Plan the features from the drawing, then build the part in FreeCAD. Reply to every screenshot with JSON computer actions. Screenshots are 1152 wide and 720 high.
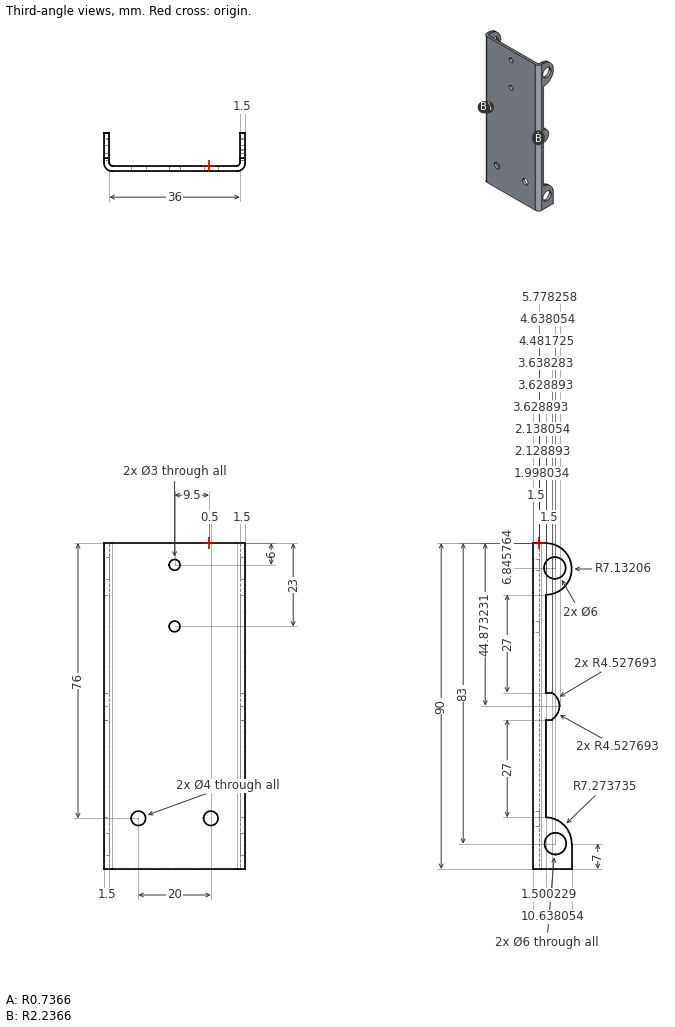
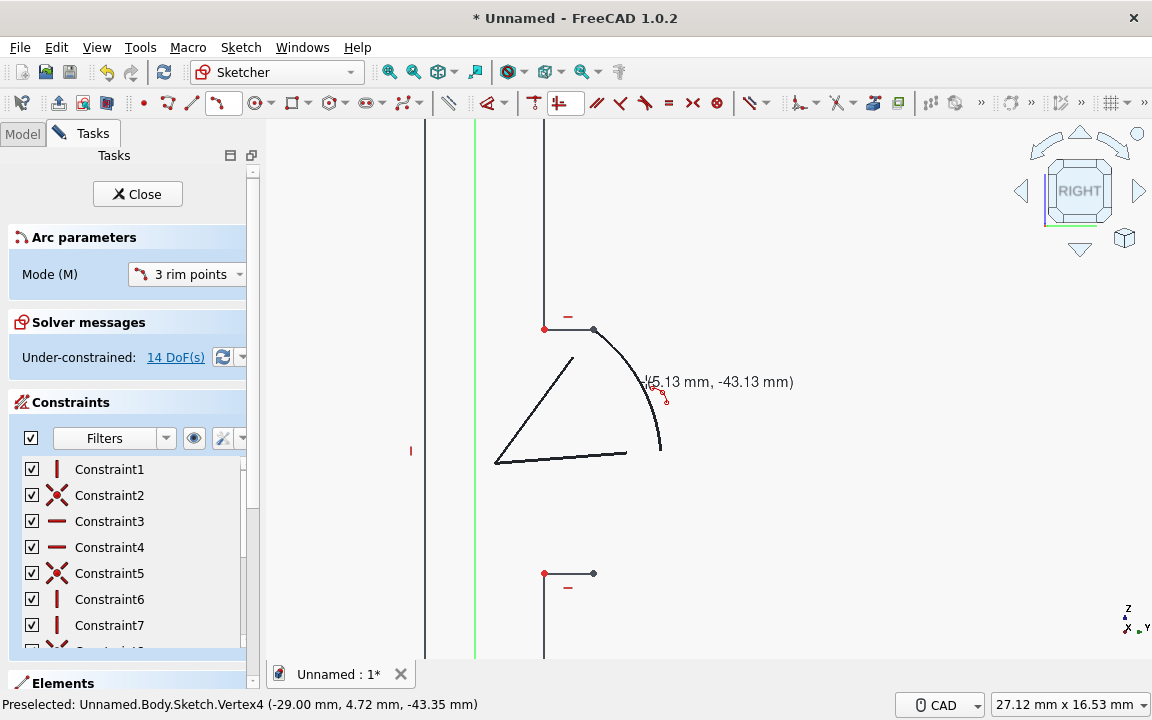
{"action": "left_click", "coordinate": [643, 376]}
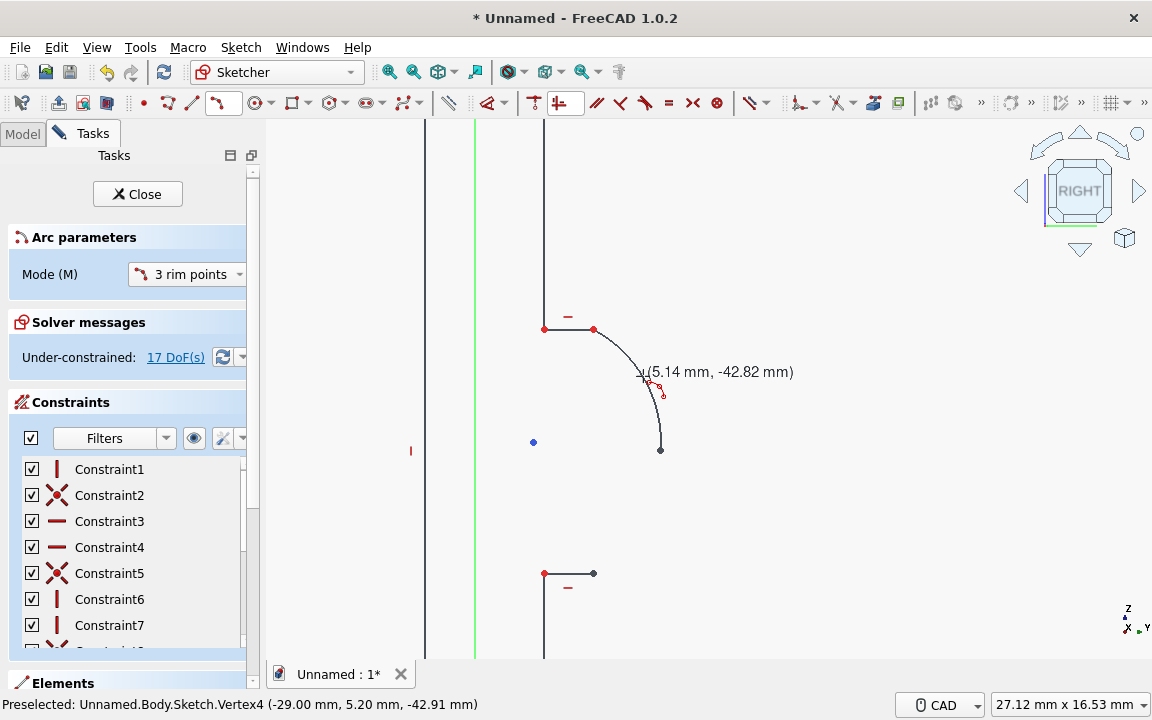
{"action": "scroll", "coordinate": [646, 382], "scroll_direction": "down", "scroll_amount": 11}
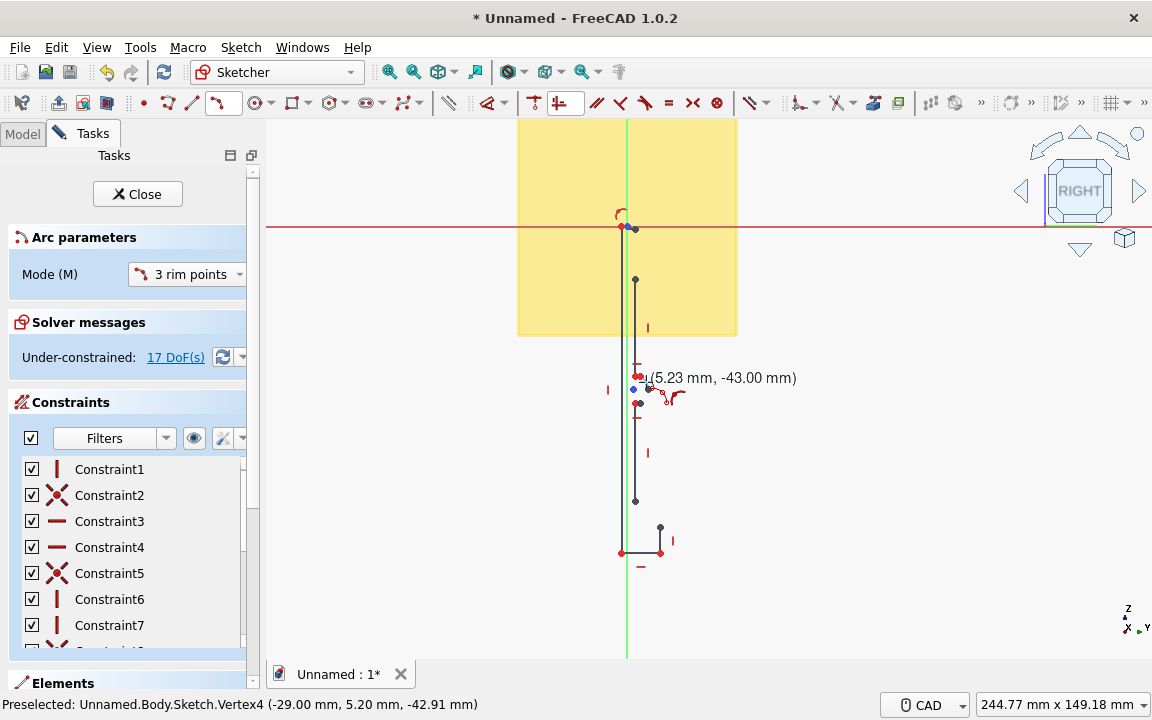
{"action": "left_click", "coordinate": [648, 390]}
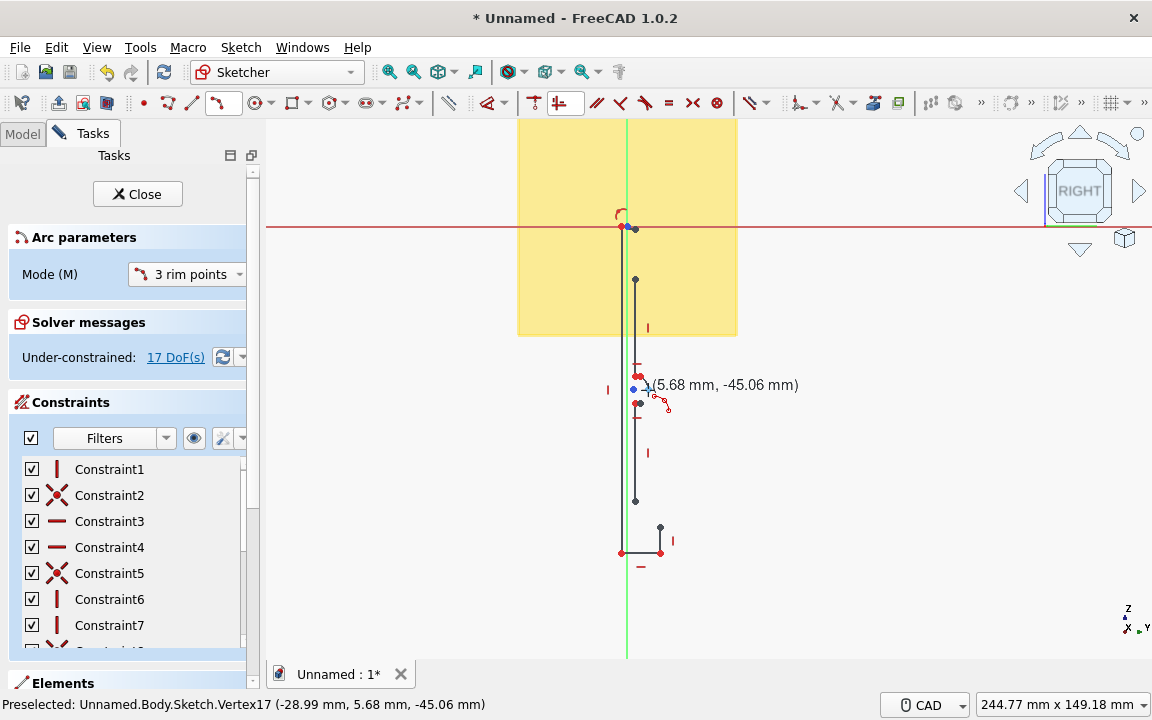
{"action": "scroll", "coordinate": [641, 403], "scroll_direction": "up", "scroll_amount": 9}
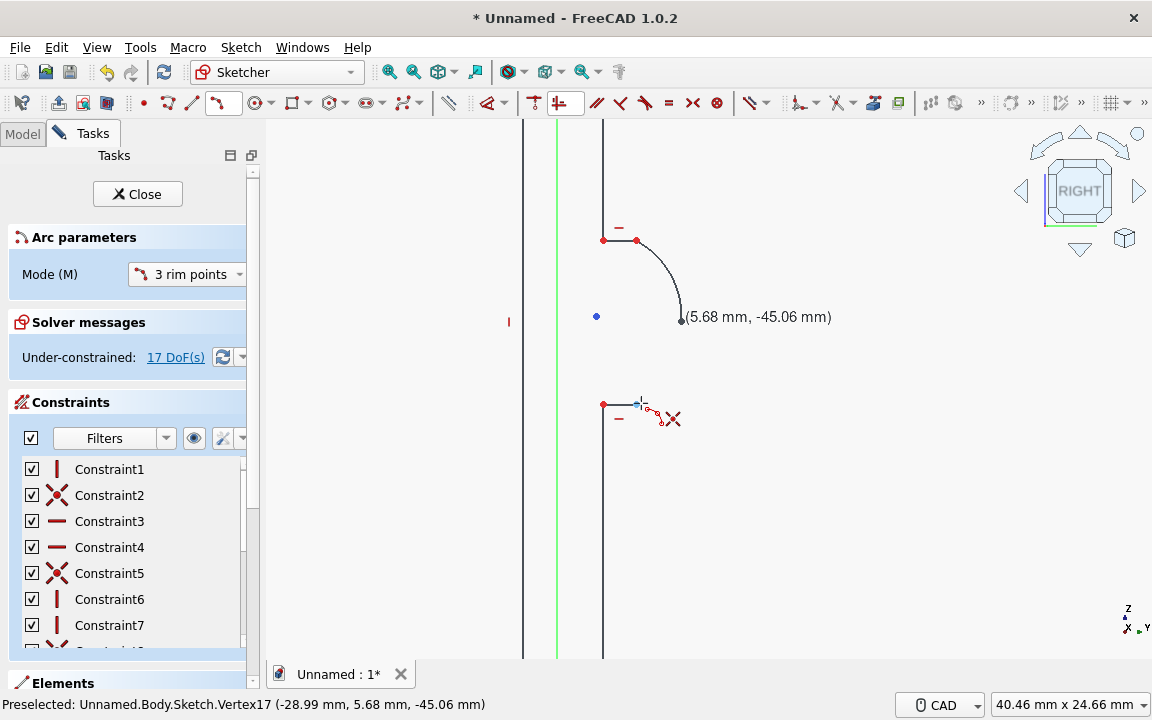
{"action": "left_click", "coordinate": [636, 405]}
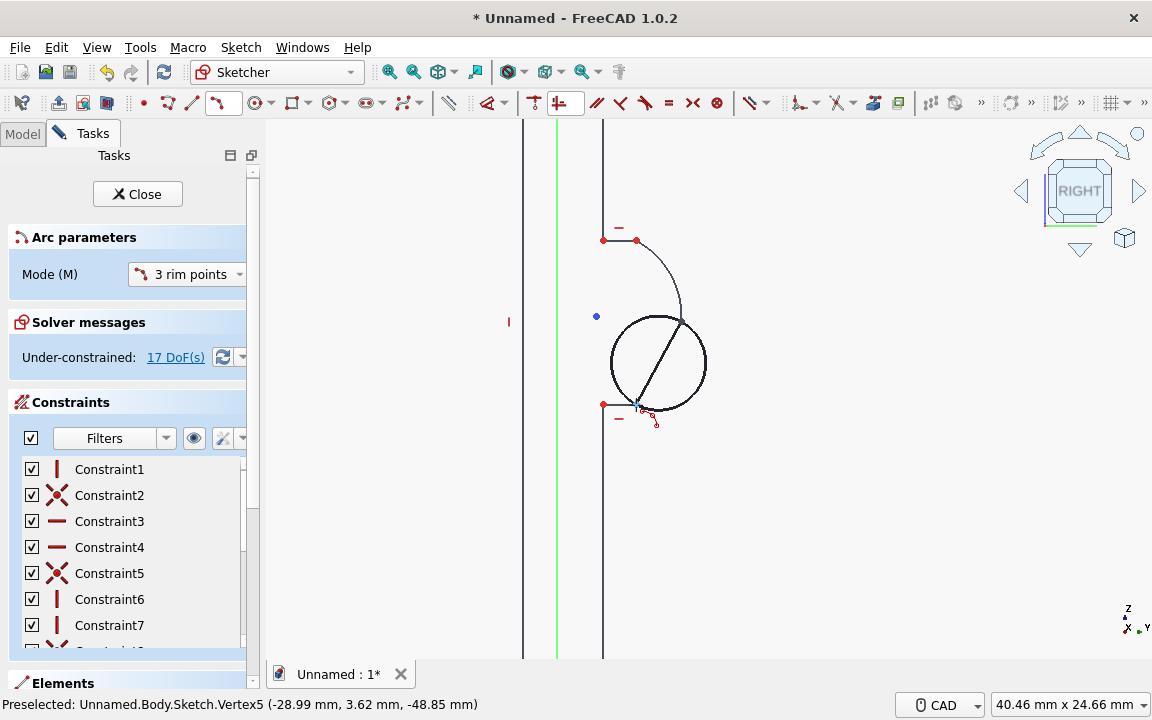
{"action": "scroll", "coordinate": [671, 366], "scroll_direction": "up", "scroll_amount": 2}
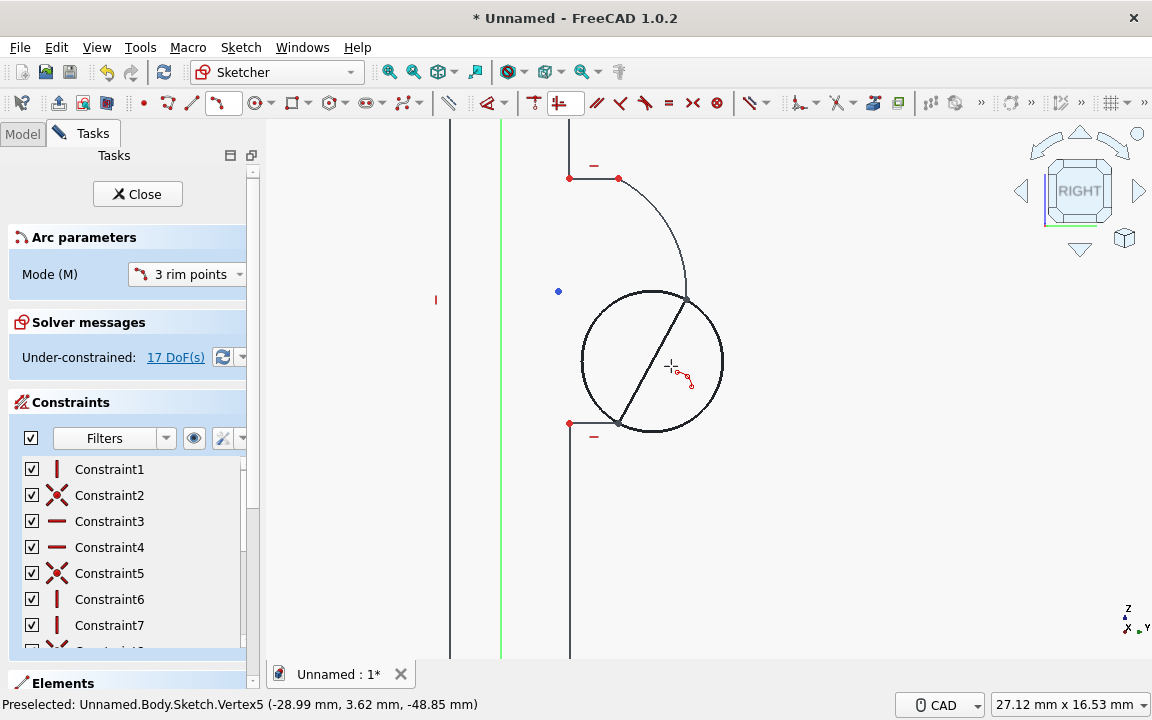
{"action": "left_click", "coordinate": [671, 366]}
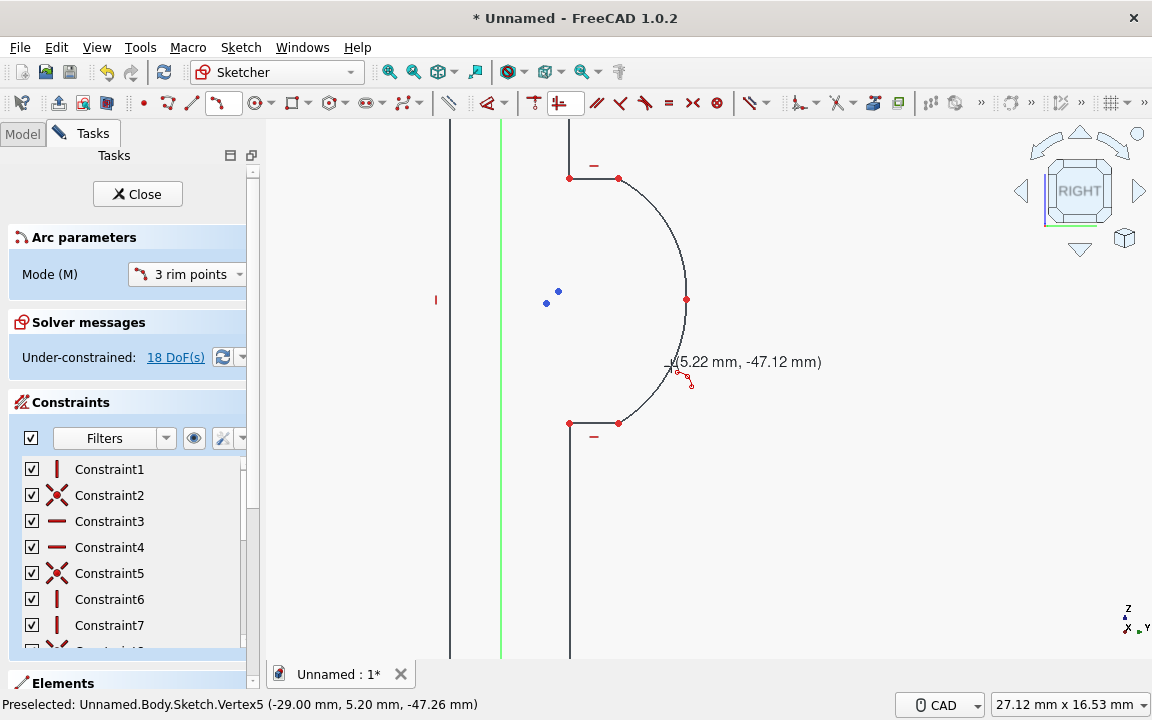
{"action": "scroll", "coordinate": [642, 400], "scroll_direction": "down", "scroll_amount": 11}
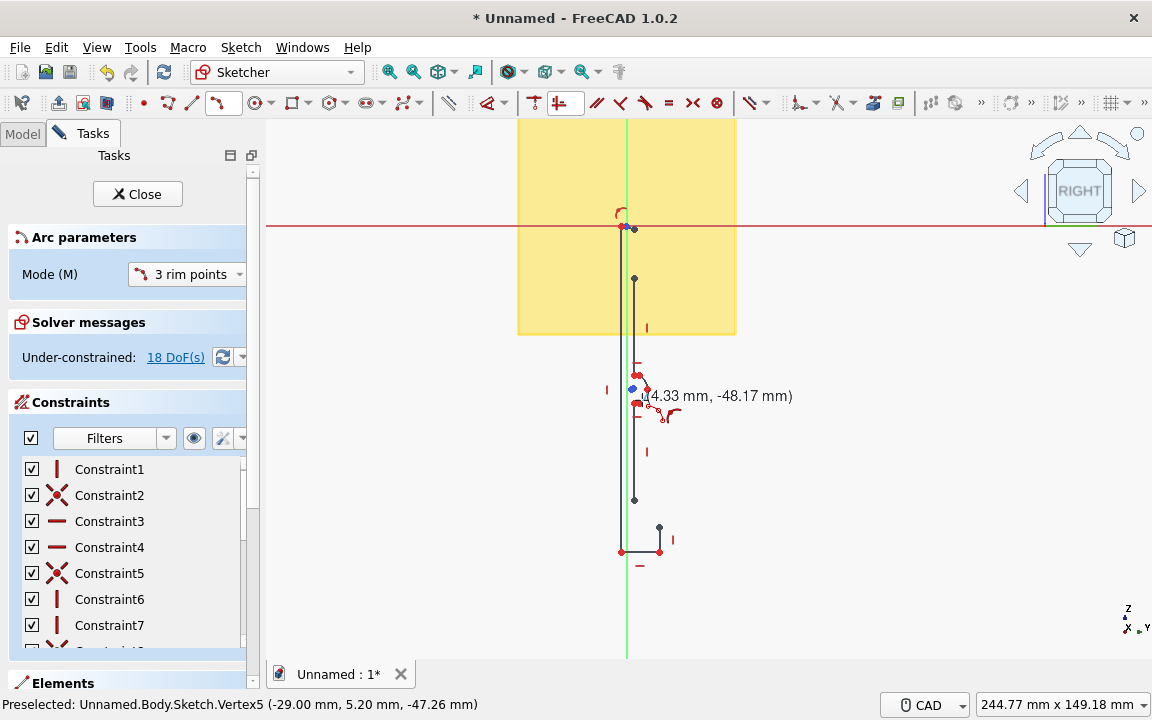
{"action": "scroll", "coordinate": [634, 500], "scroll_direction": "up", "scroll_amount": 4}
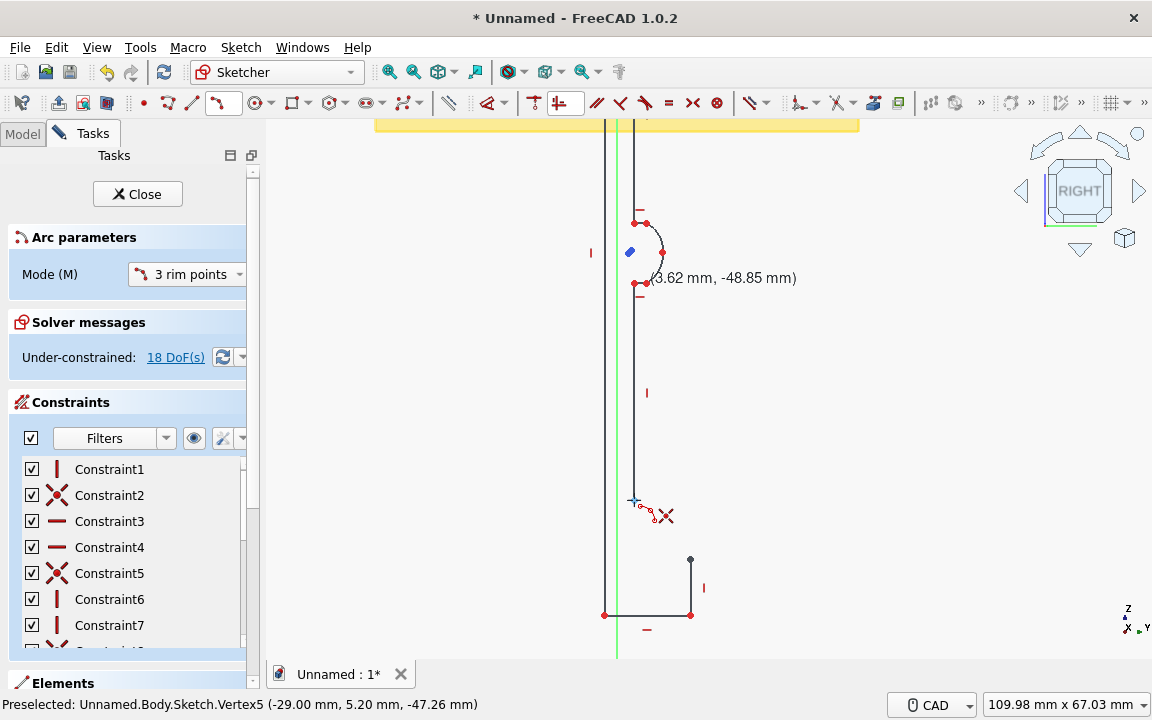
{"action": "left_click", "coordinate": [634, 501]}
{"action": "left_click", "coordinate": [691, 560]}
{"action": "left_click", "coordinate": [674, 518]}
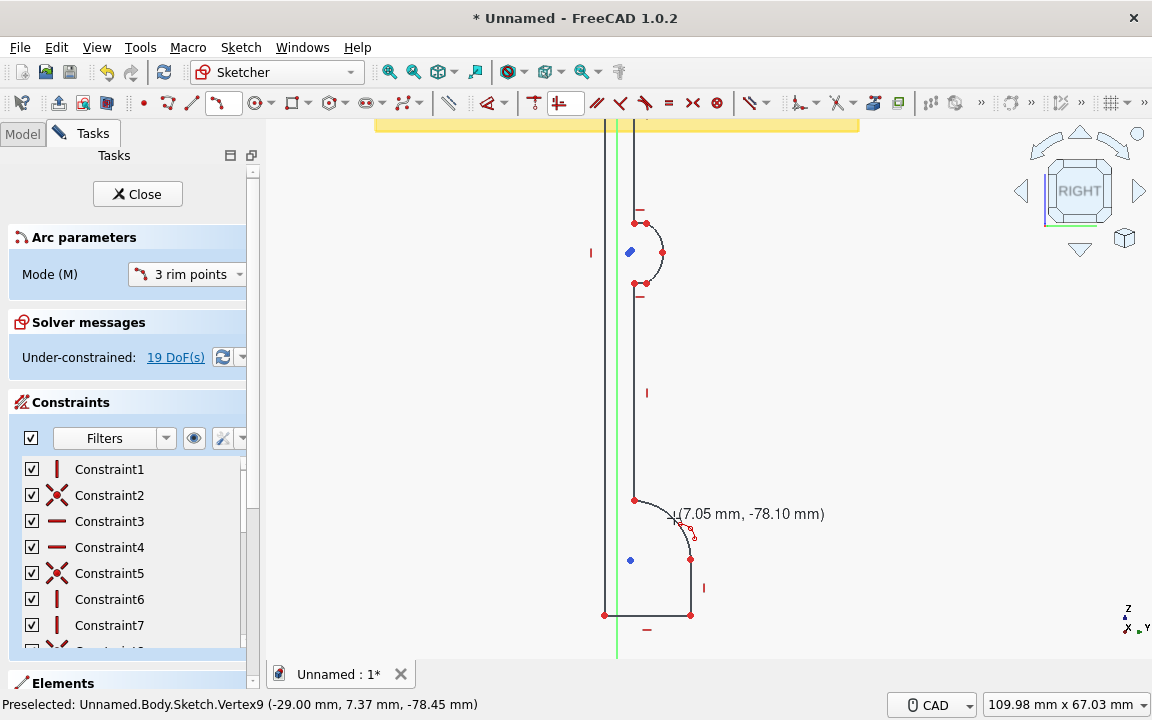
{"action": "scroll", "coordinate": [634, 500], "scroll_direction": "down", "scroll_amount": 4}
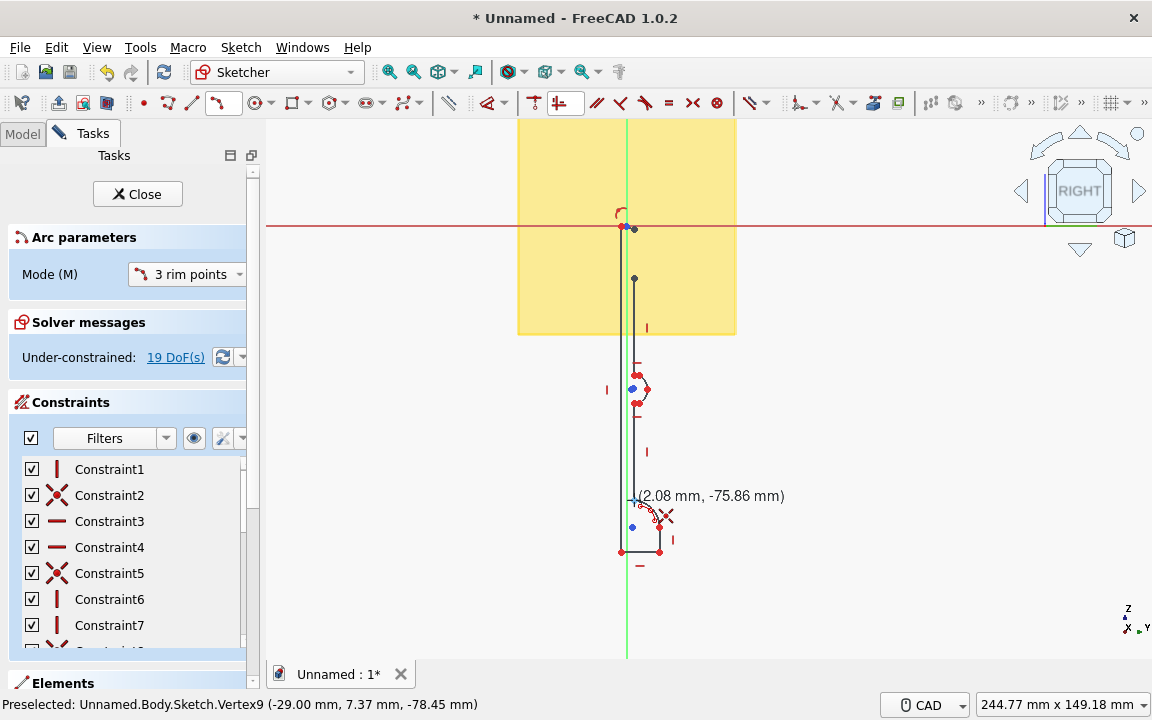
{"action": "scroll", "coordinate": [634, 226], "scroll_direction": "up", "scroll_amount": 5}